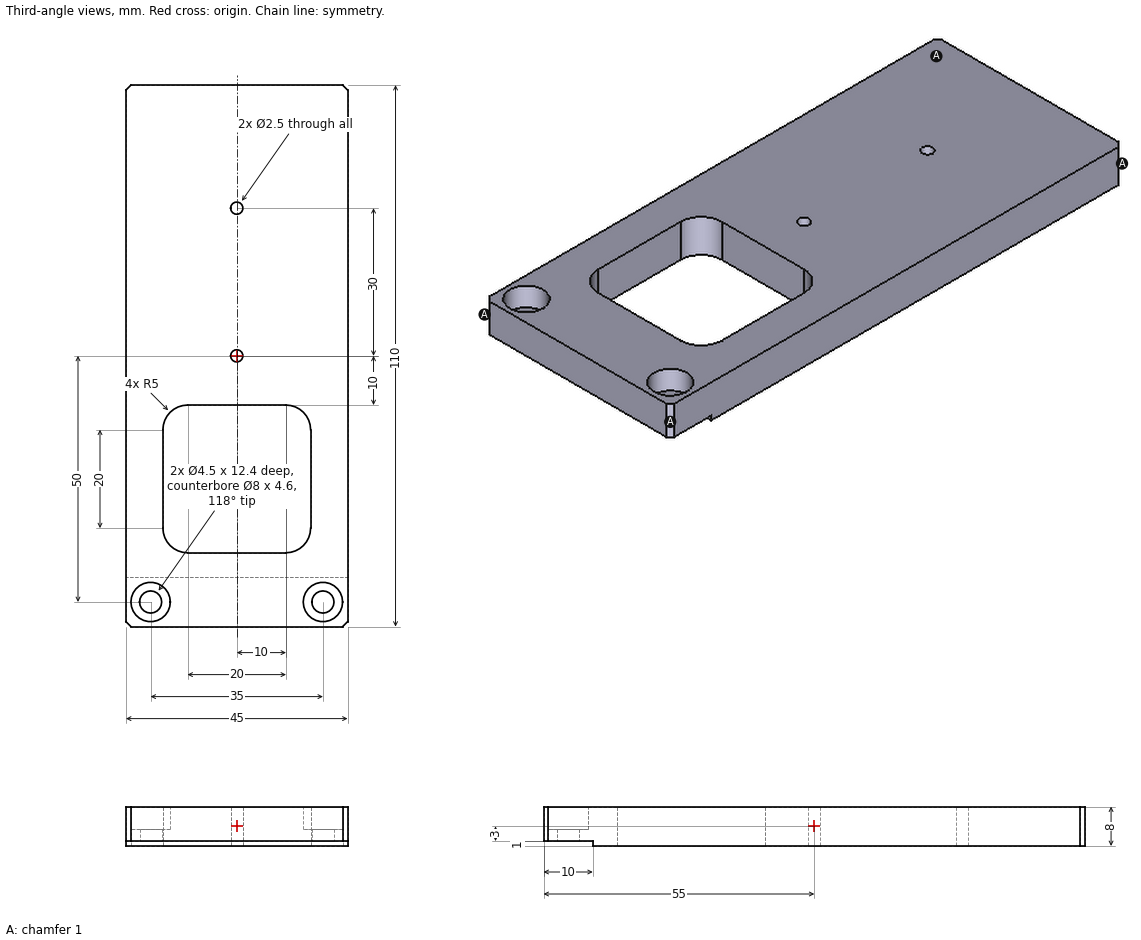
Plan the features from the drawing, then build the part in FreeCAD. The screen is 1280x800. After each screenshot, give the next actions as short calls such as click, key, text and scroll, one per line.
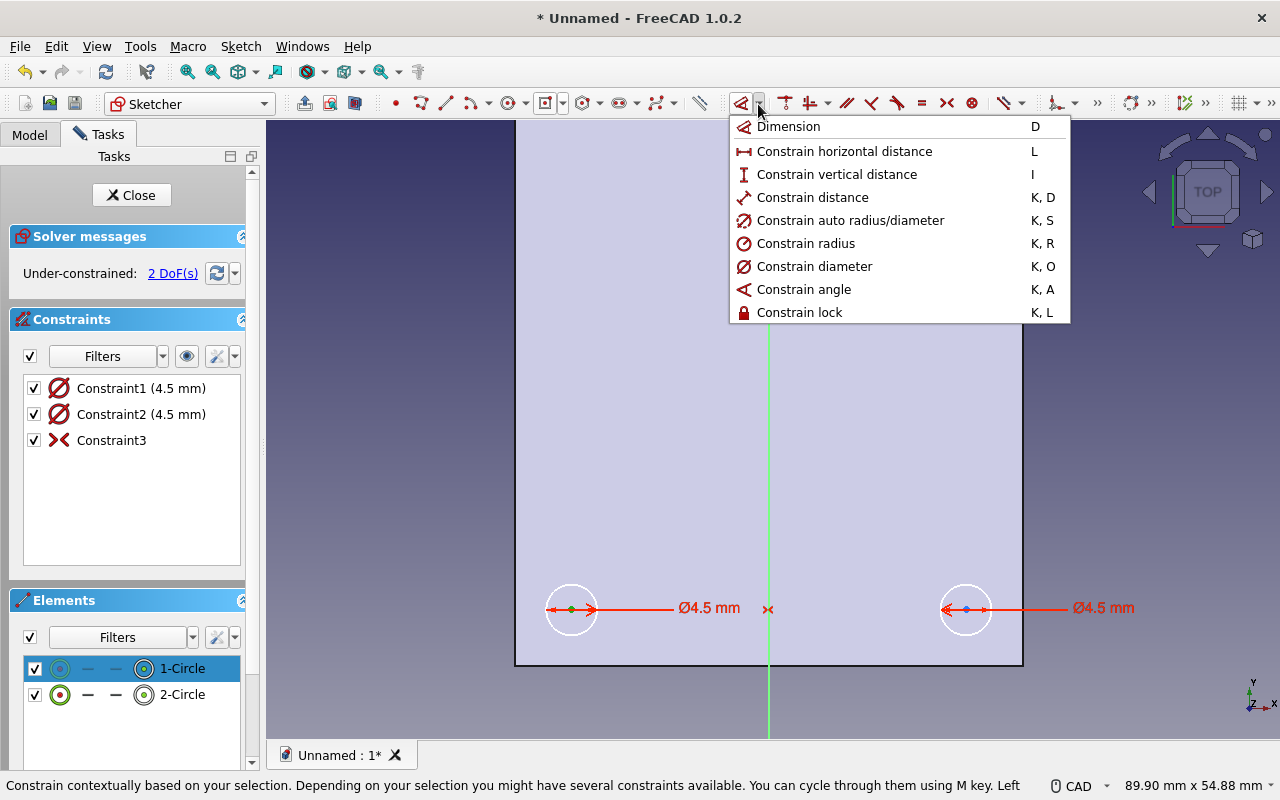
click(900, 174)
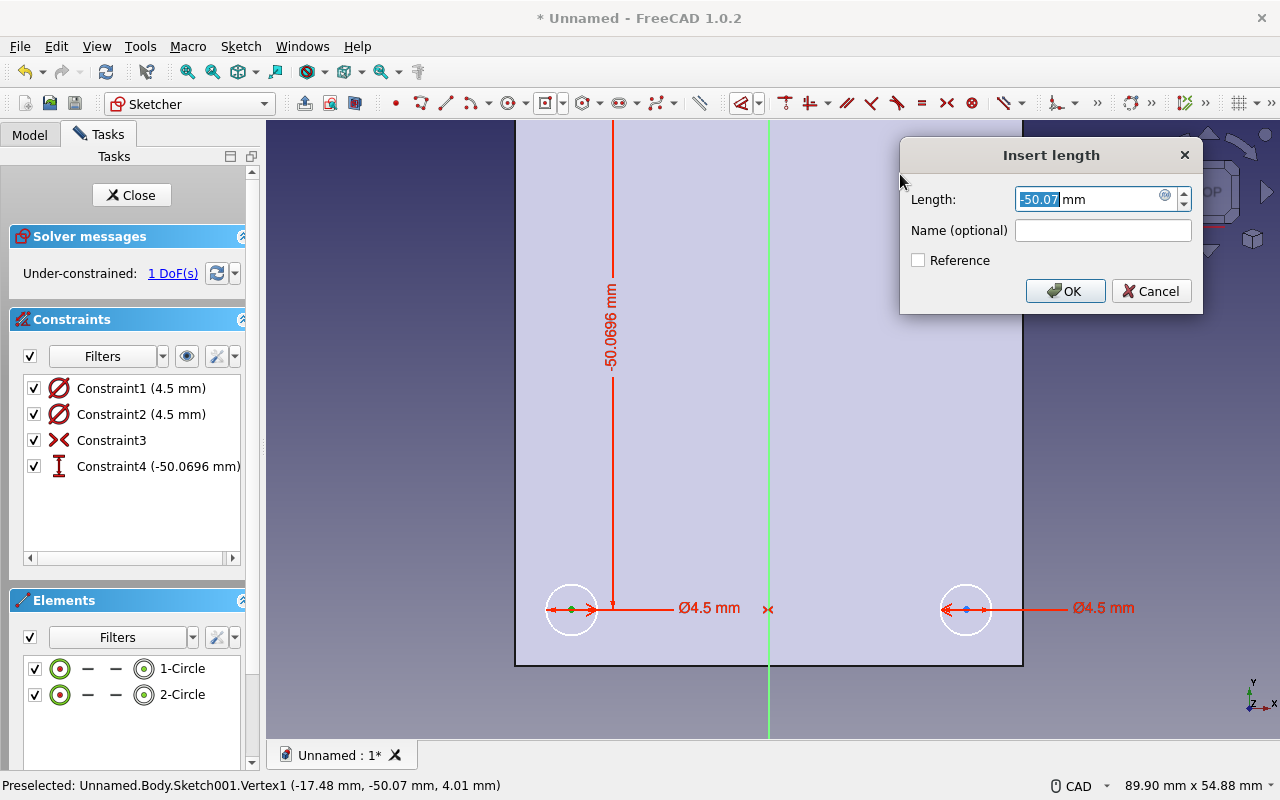
text(-50)
key(Return)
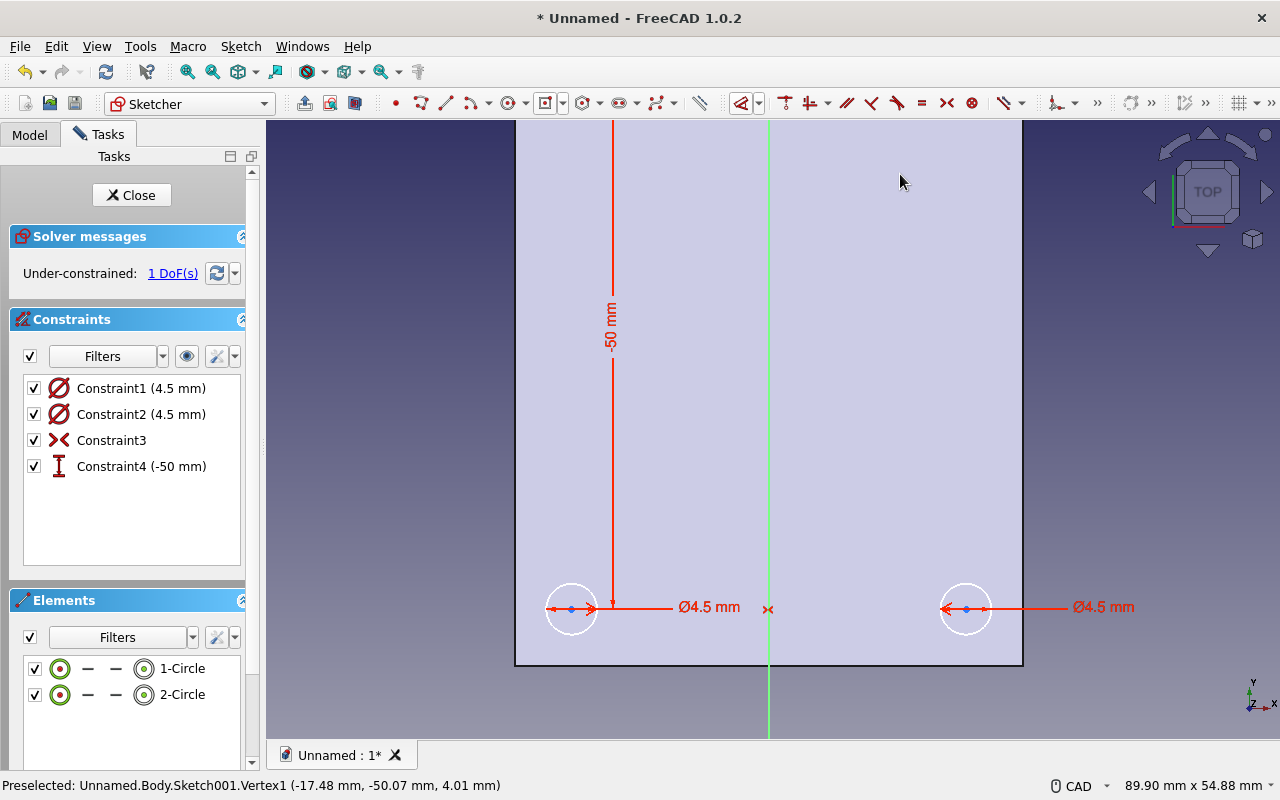
click(572, 609)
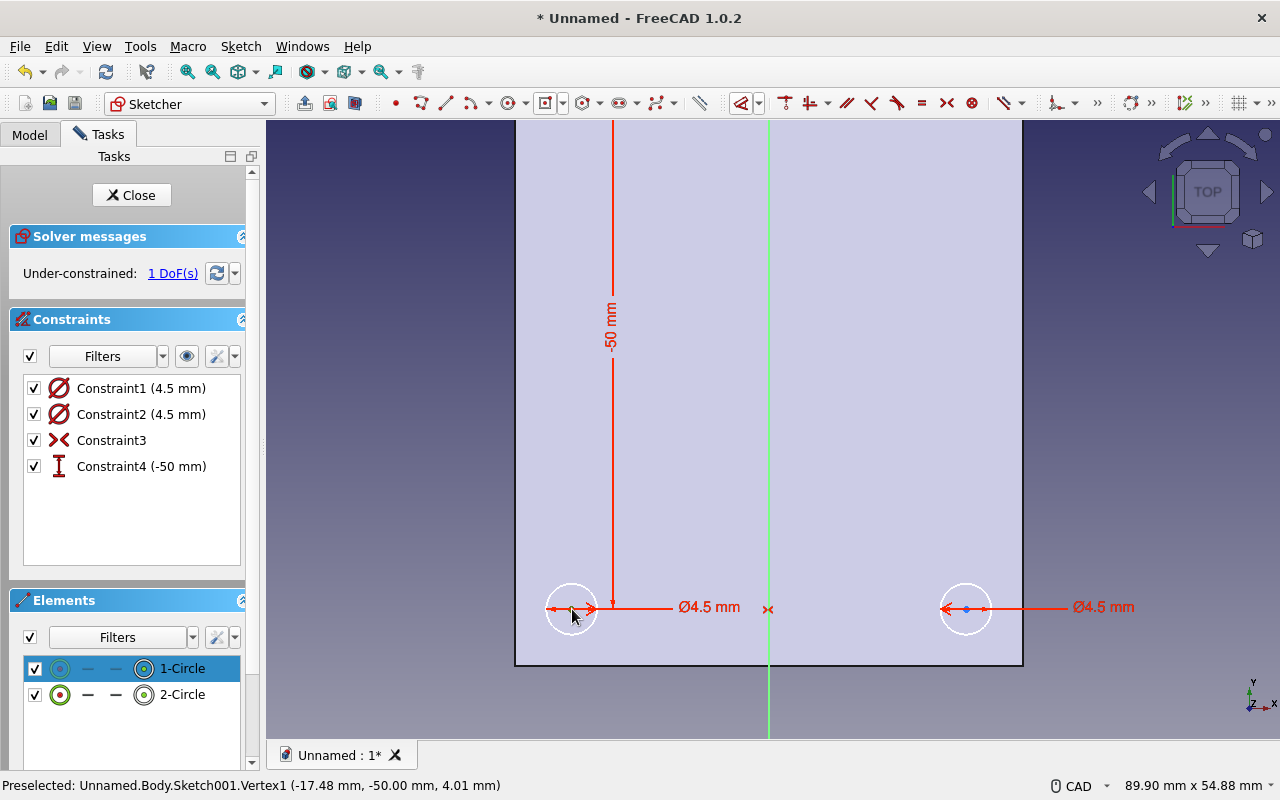
click(966, 609)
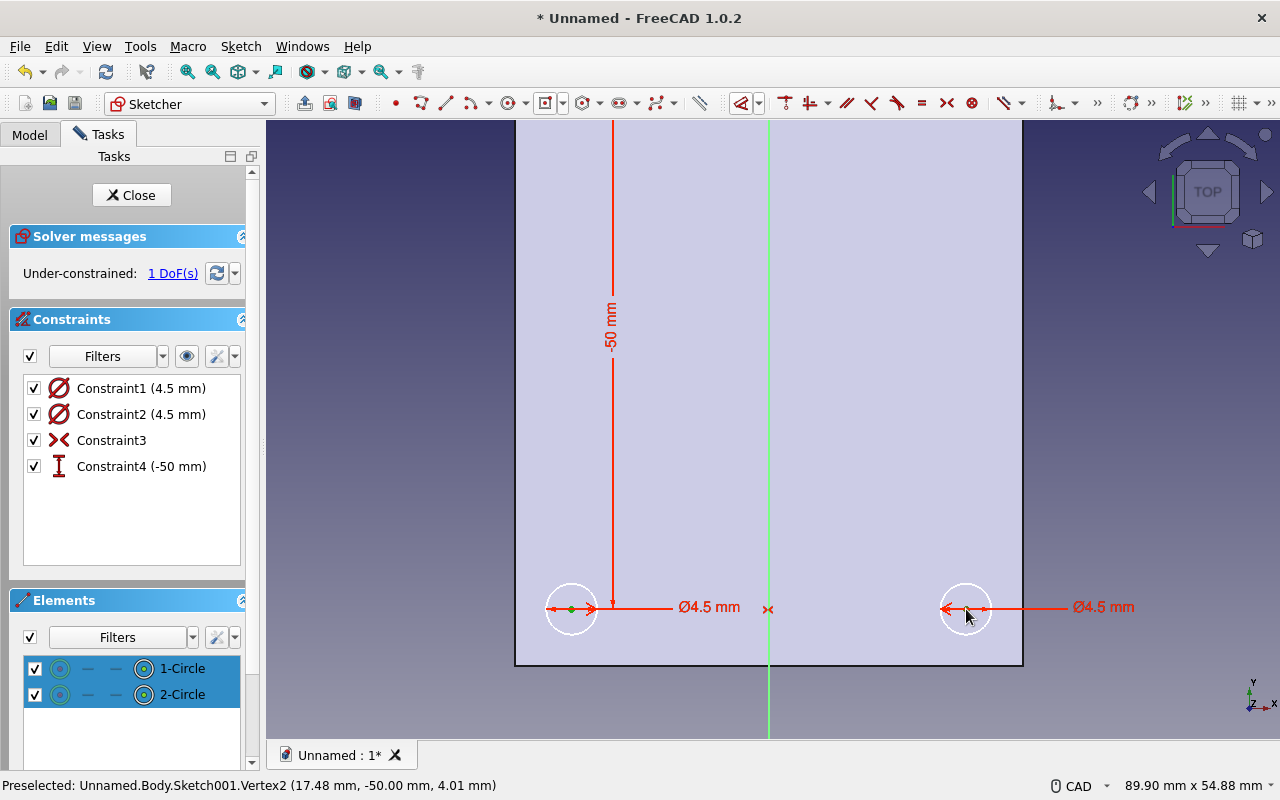
click(758, 104)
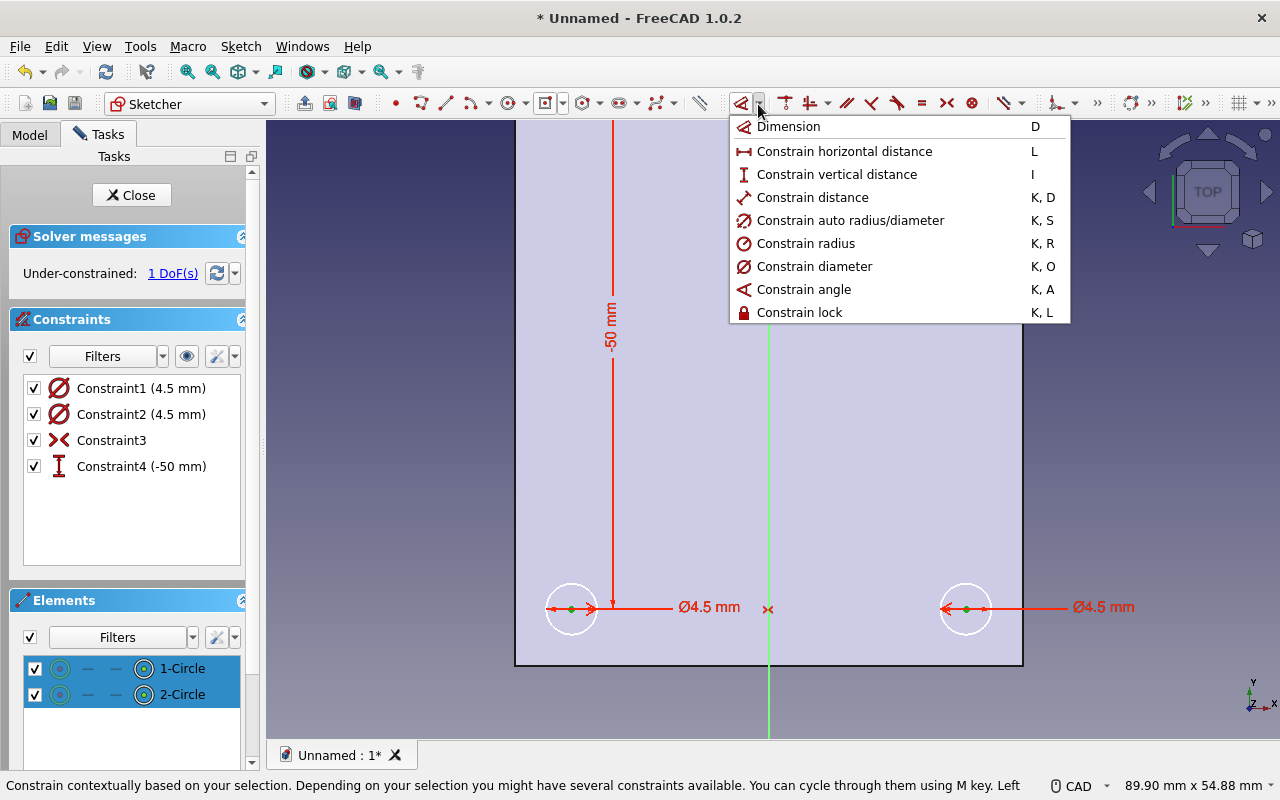
click(900, 152)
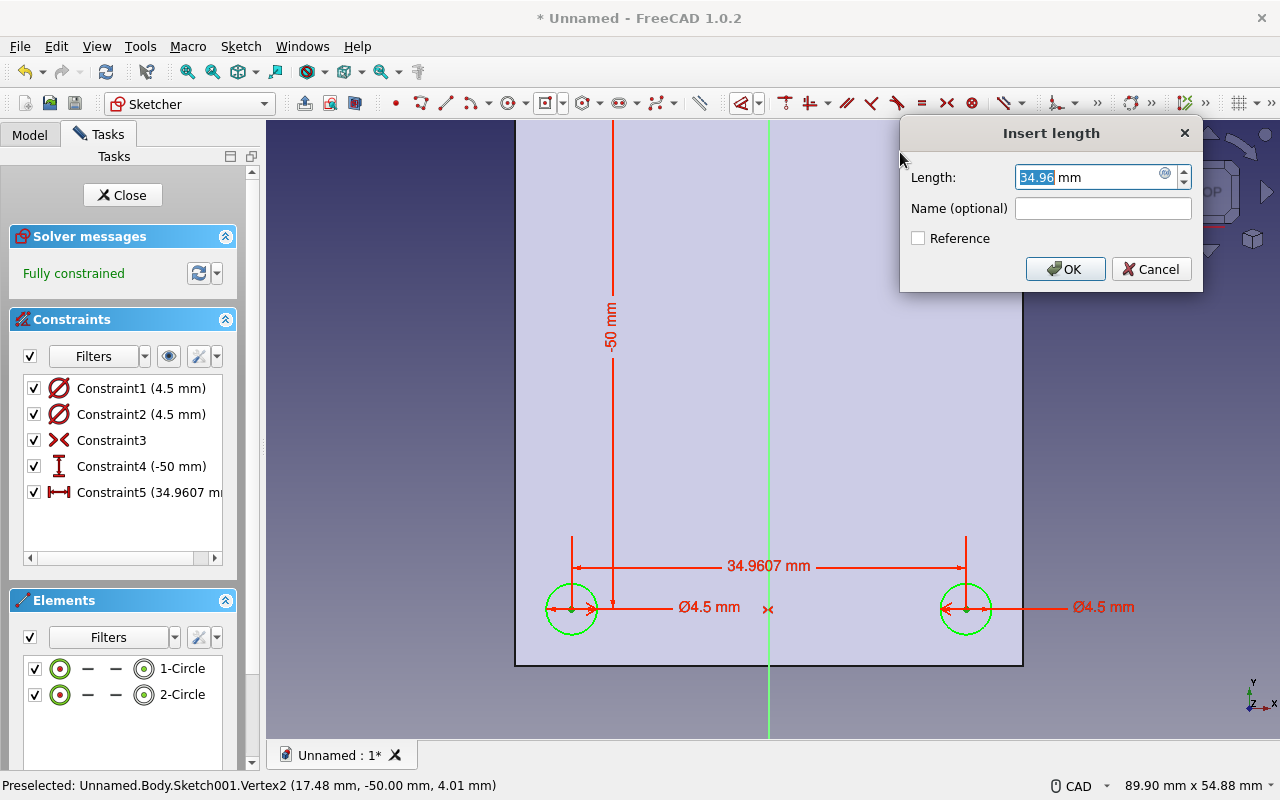
text(35)
key(Return)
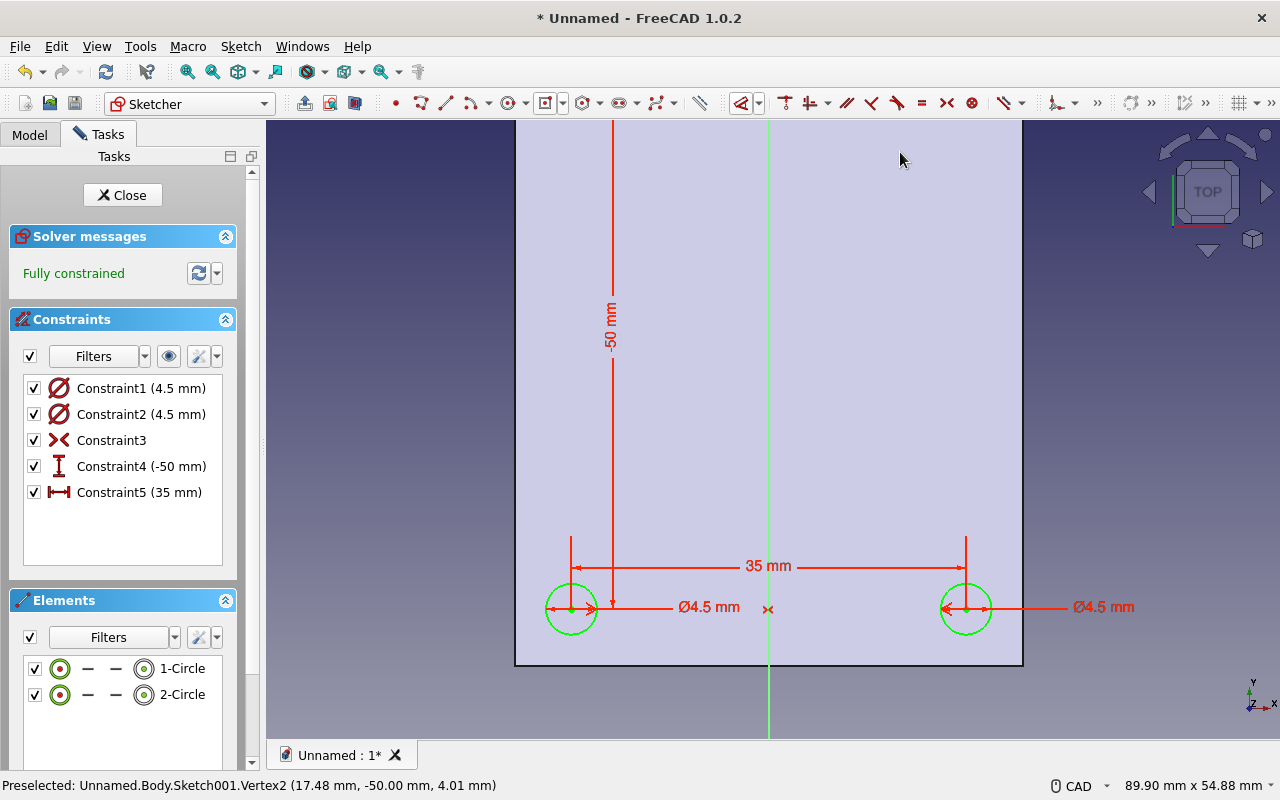
click(123, 195)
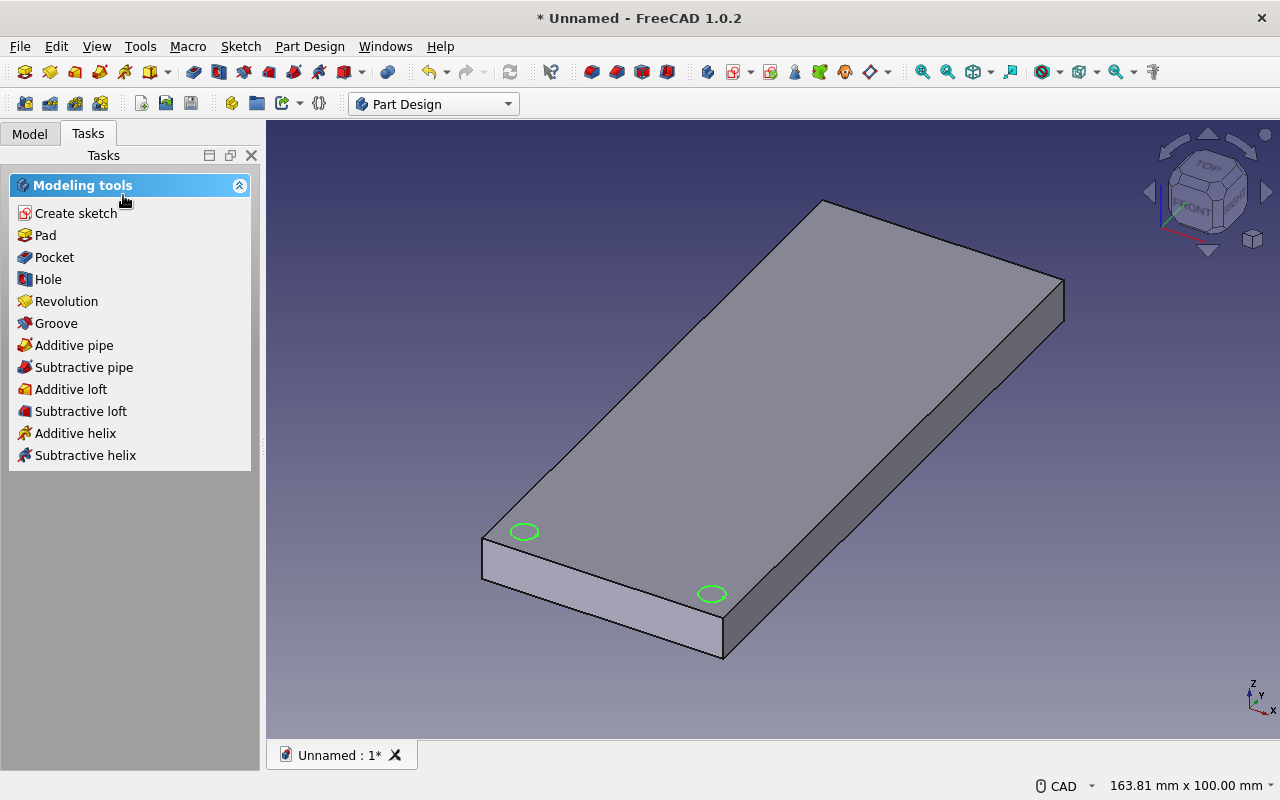
click(219, 72)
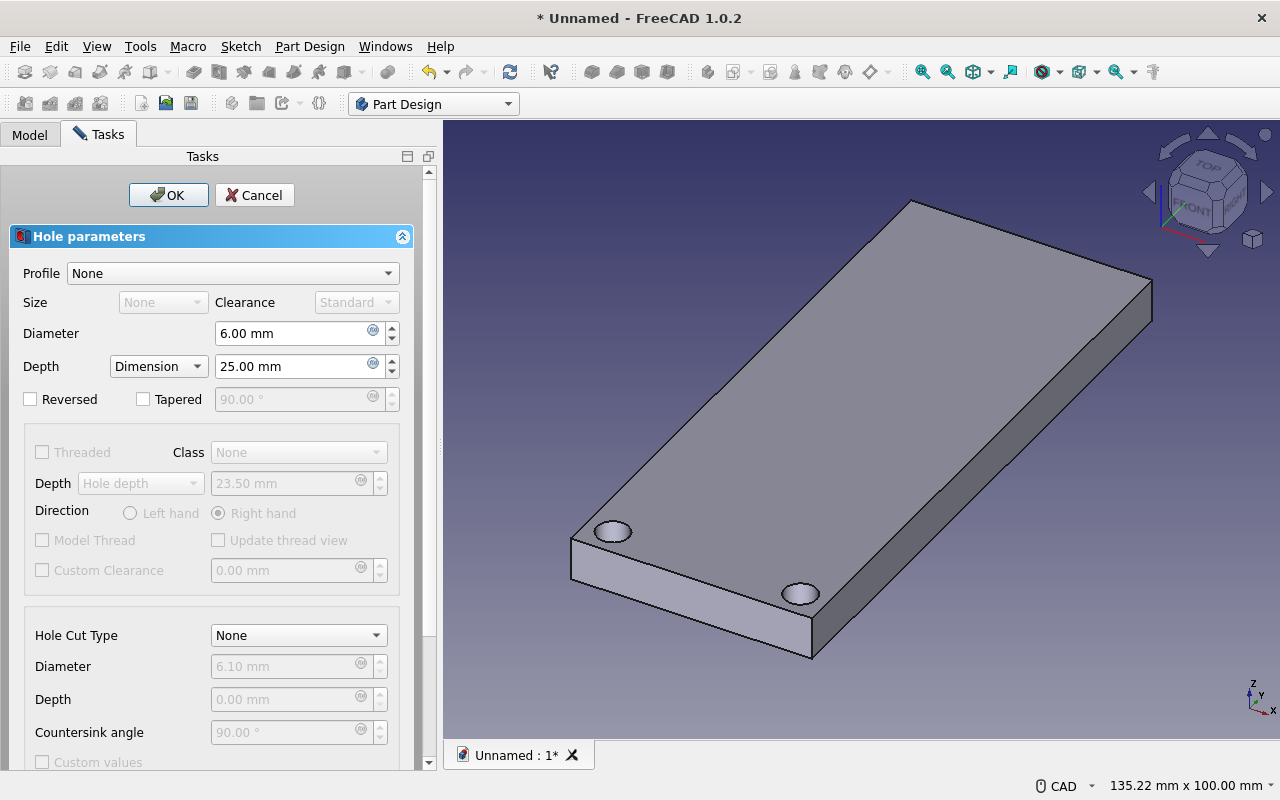
triple_click(300, 334)